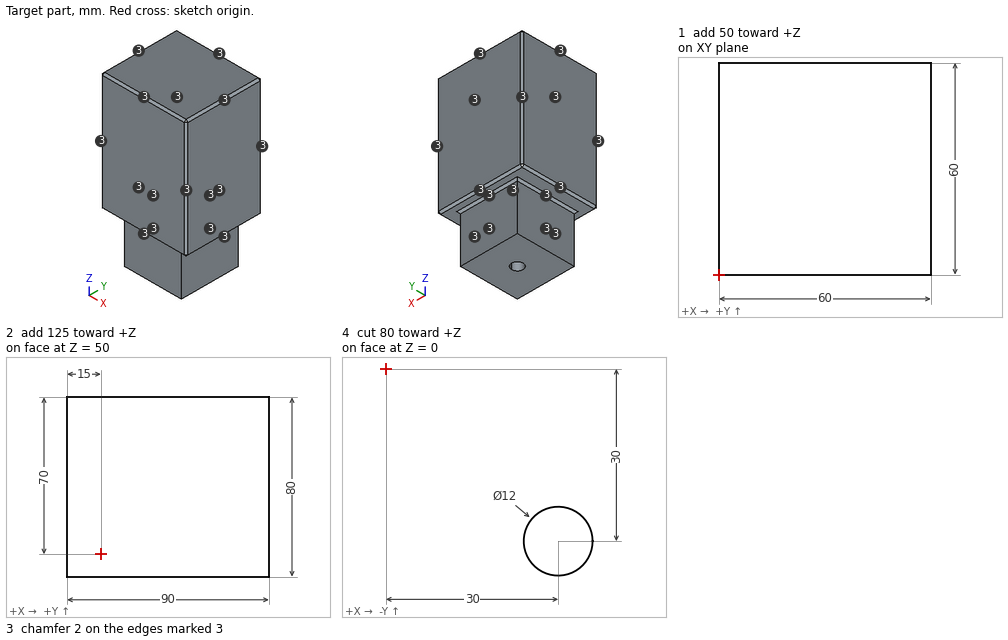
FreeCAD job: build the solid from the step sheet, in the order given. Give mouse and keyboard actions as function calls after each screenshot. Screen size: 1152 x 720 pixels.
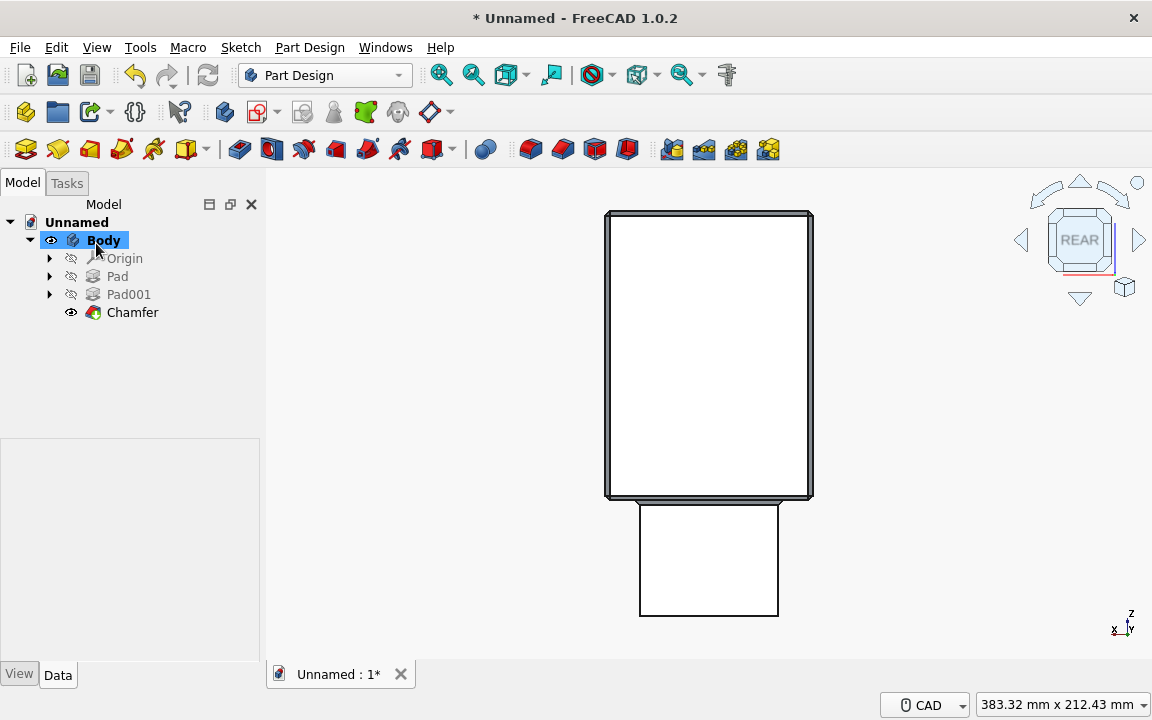
key(5)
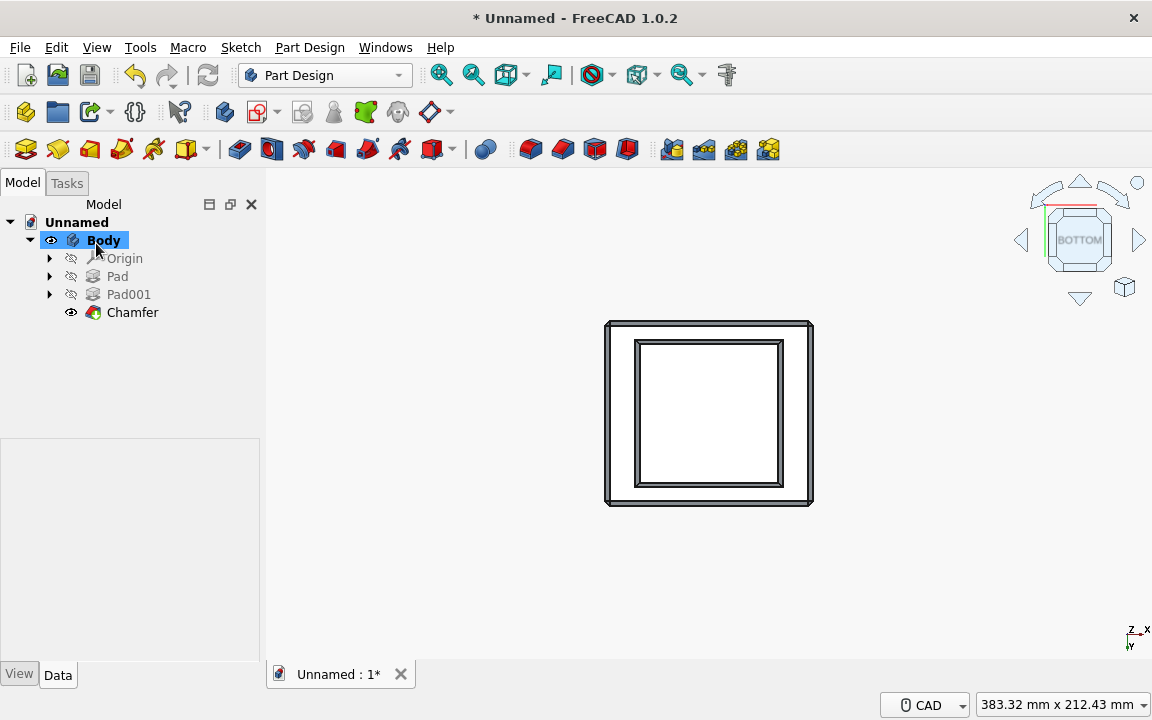
key(v)
key(f)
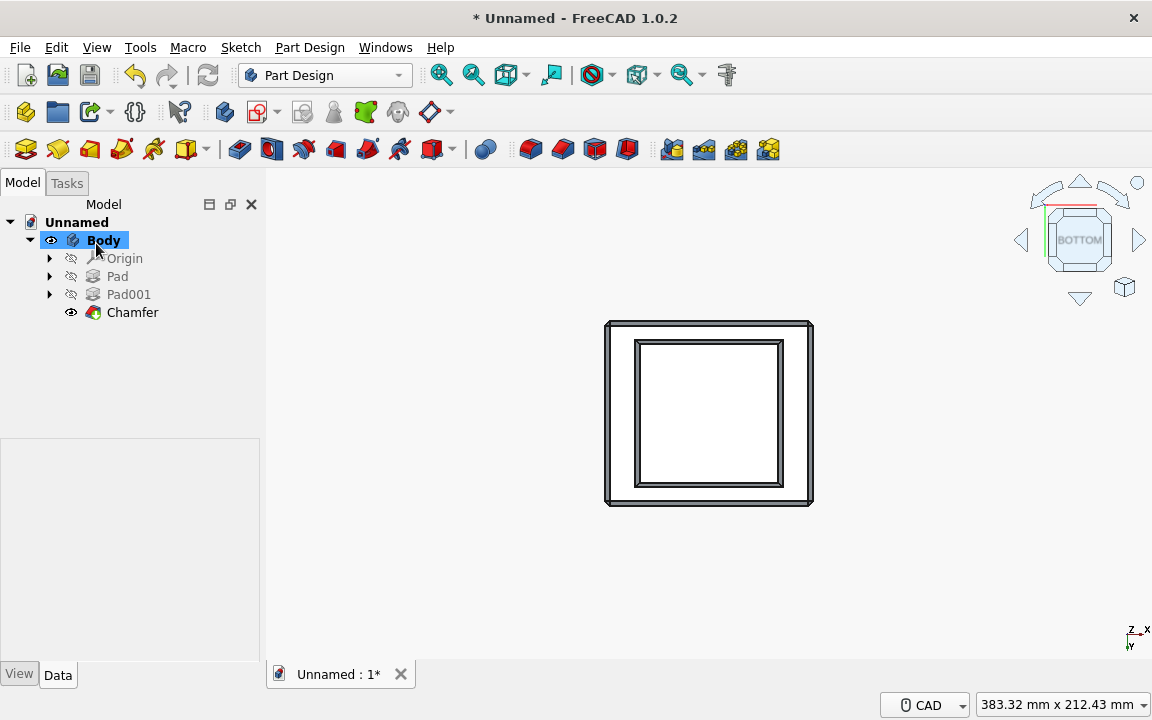
click(709, 412)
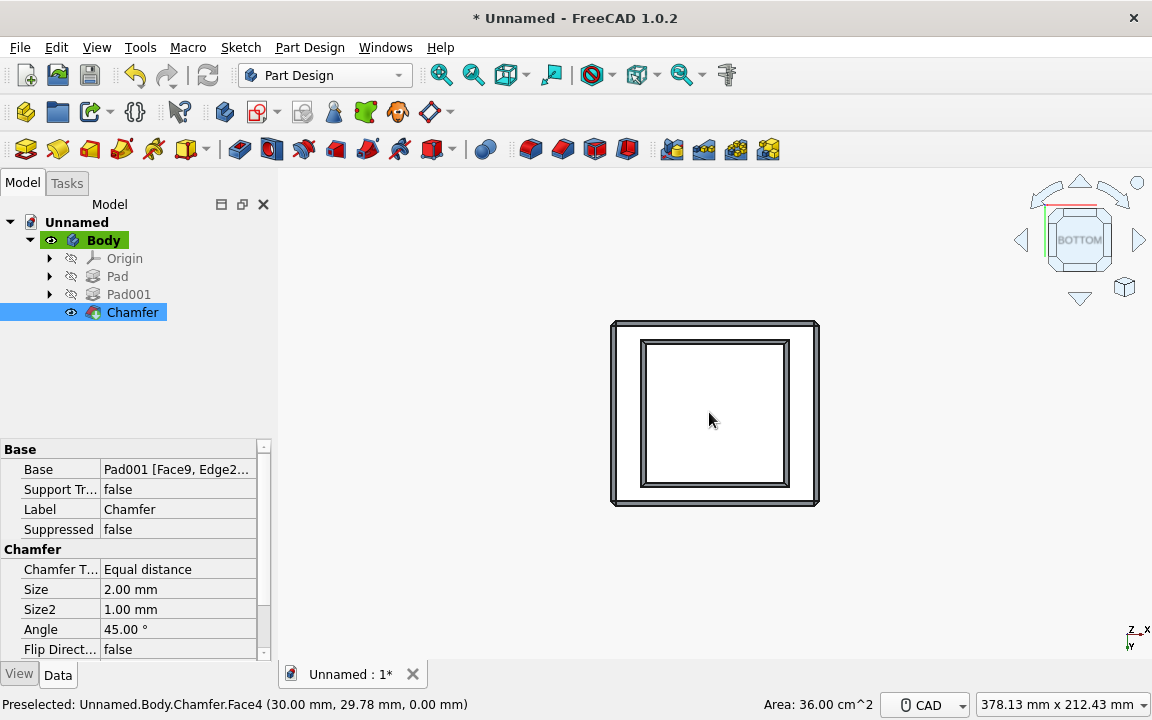
click(258, 112)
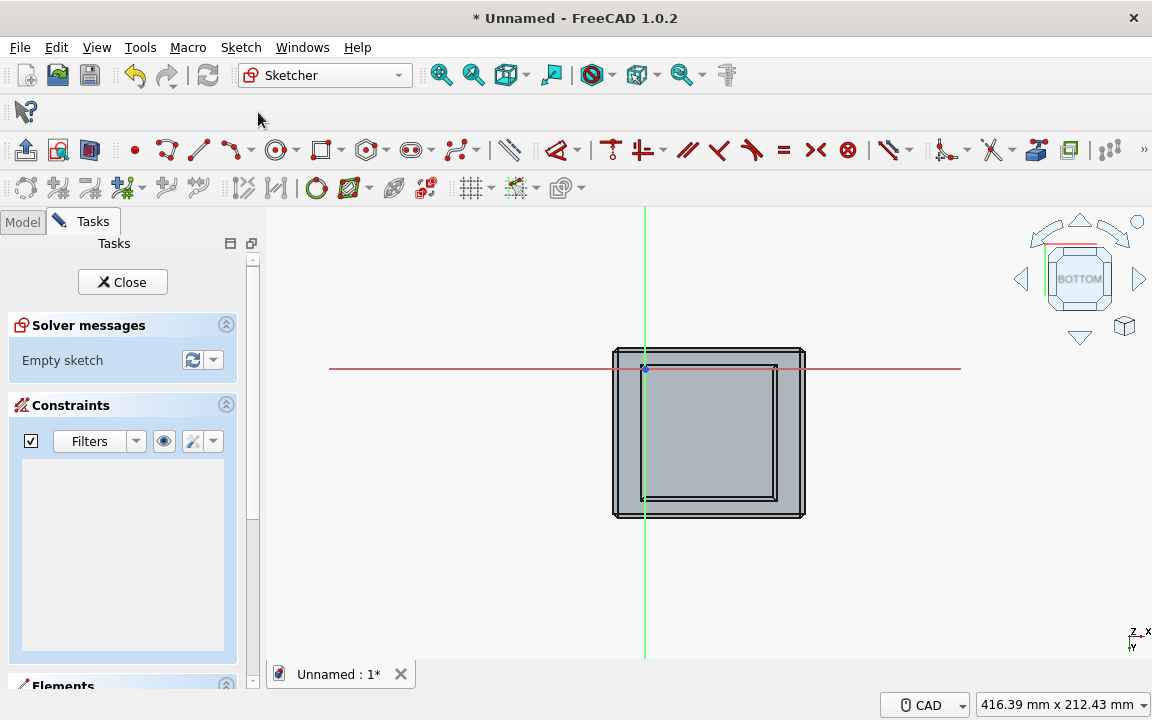
scroll(716, 433, up, 12)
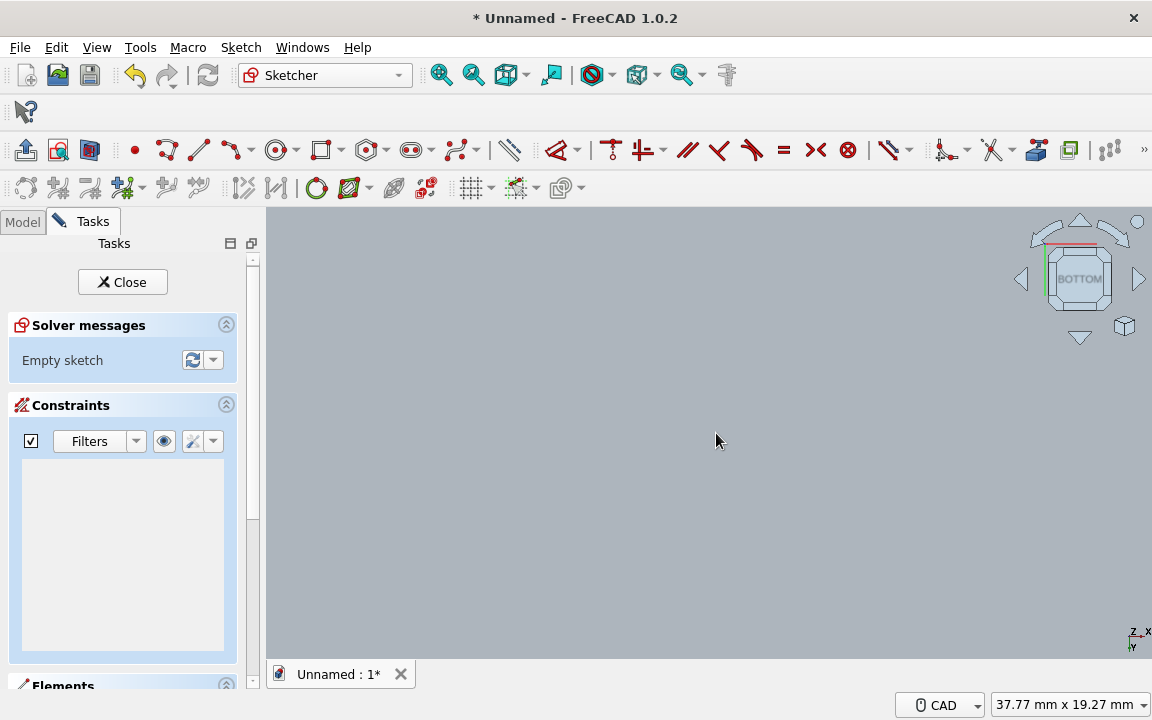
key(g)
key(c)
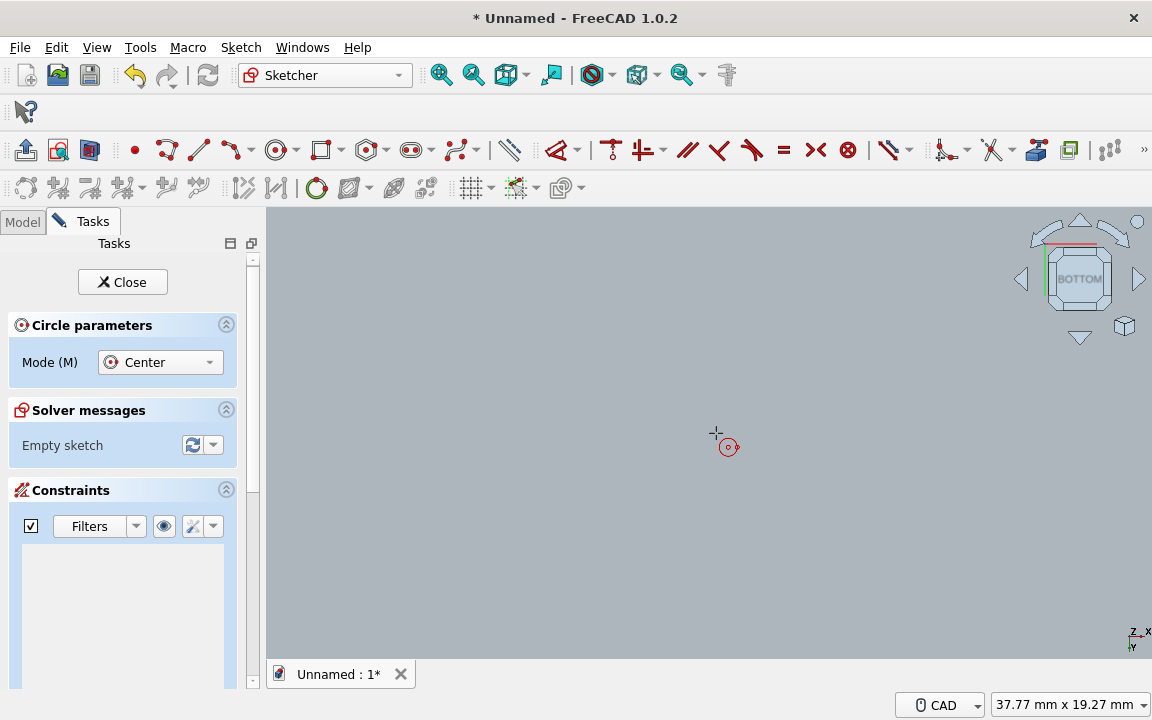
click(634, 428)
move(733, 328)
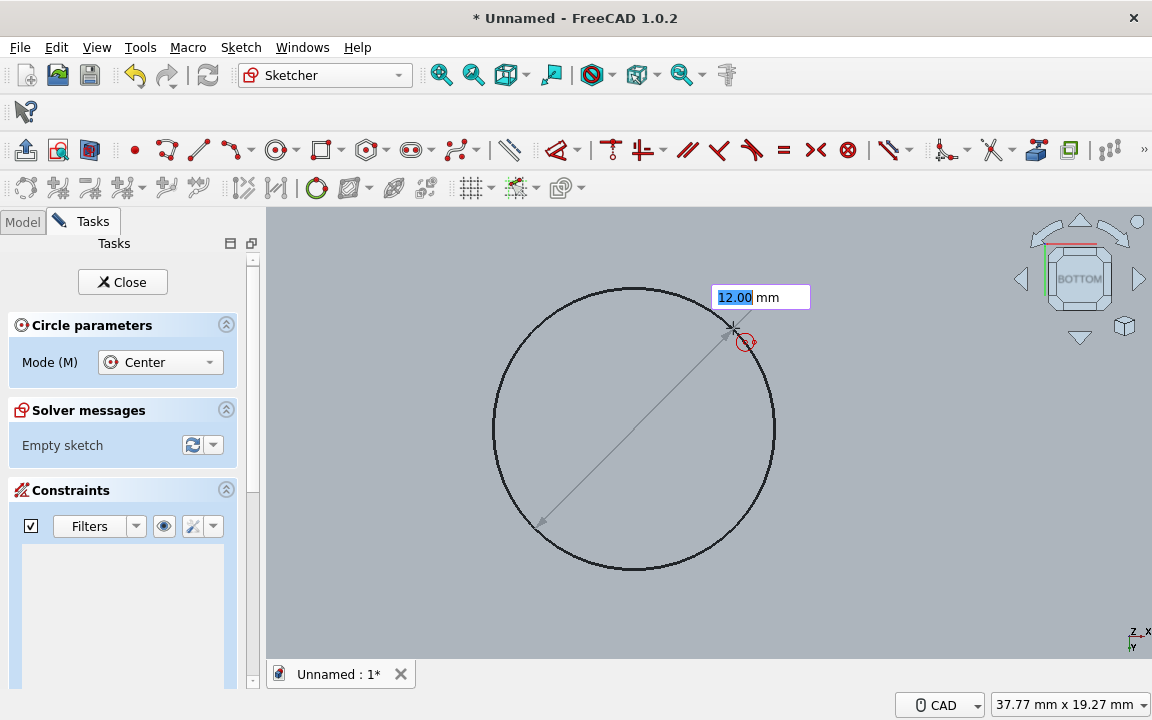
text(12)
key(Return)
key(Escape)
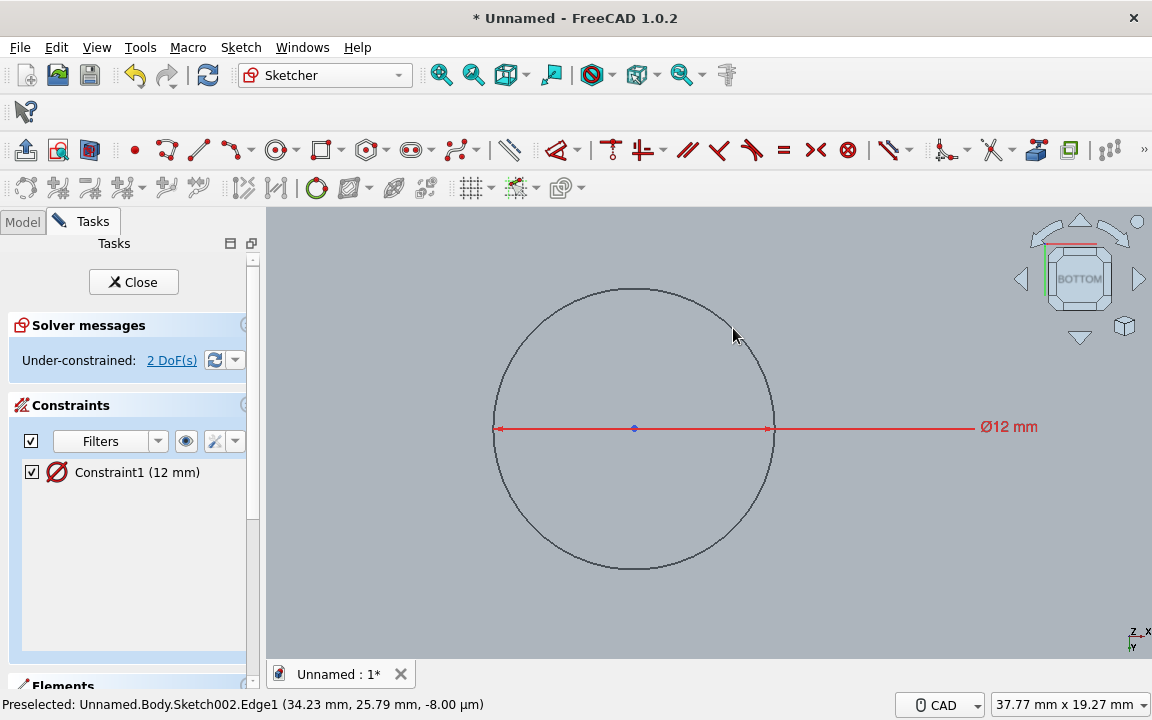
click(634, 429)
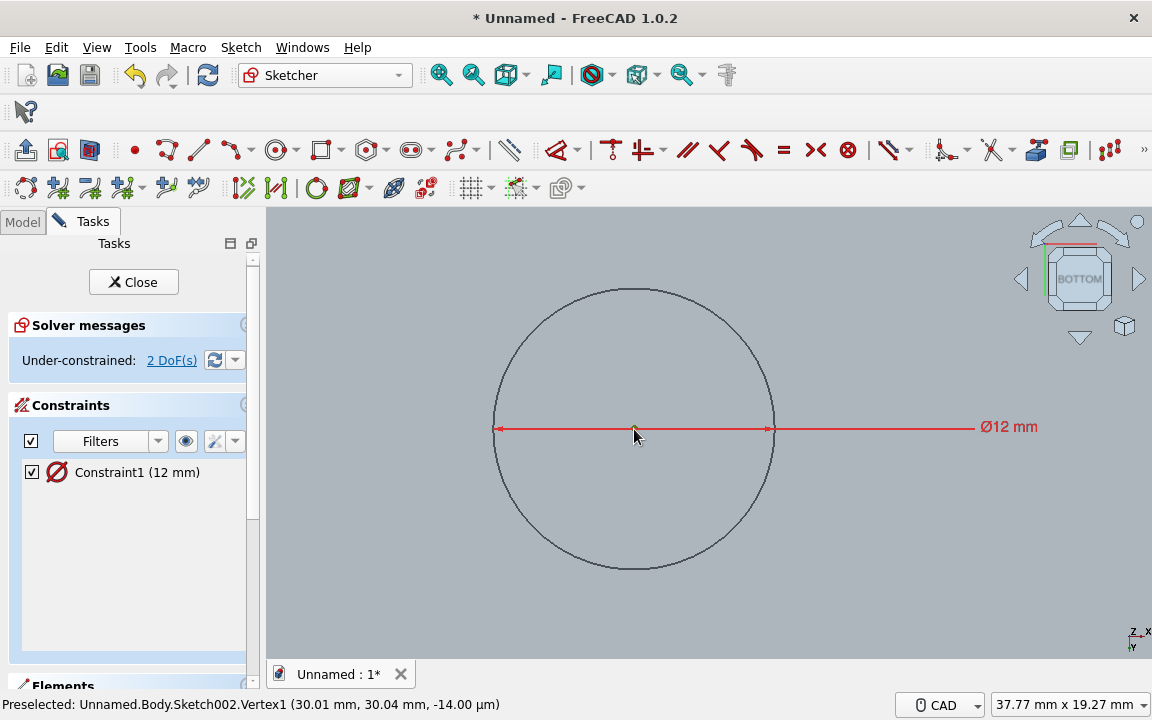
key(l)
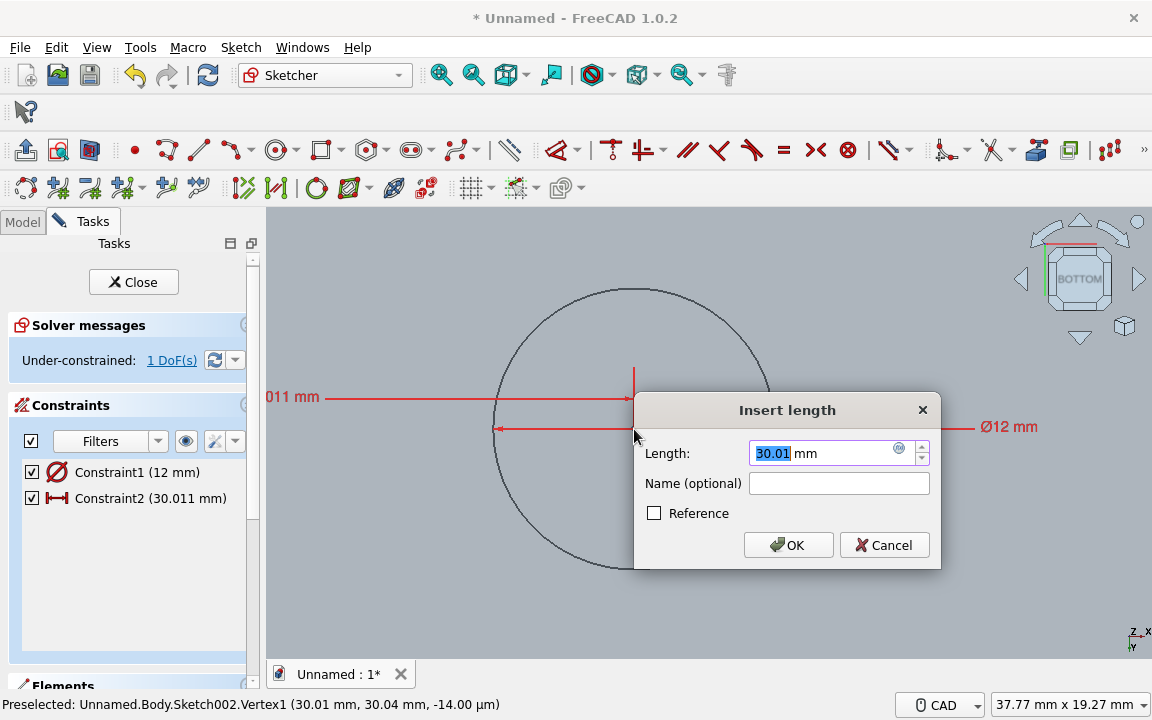
text(30)
key(Return)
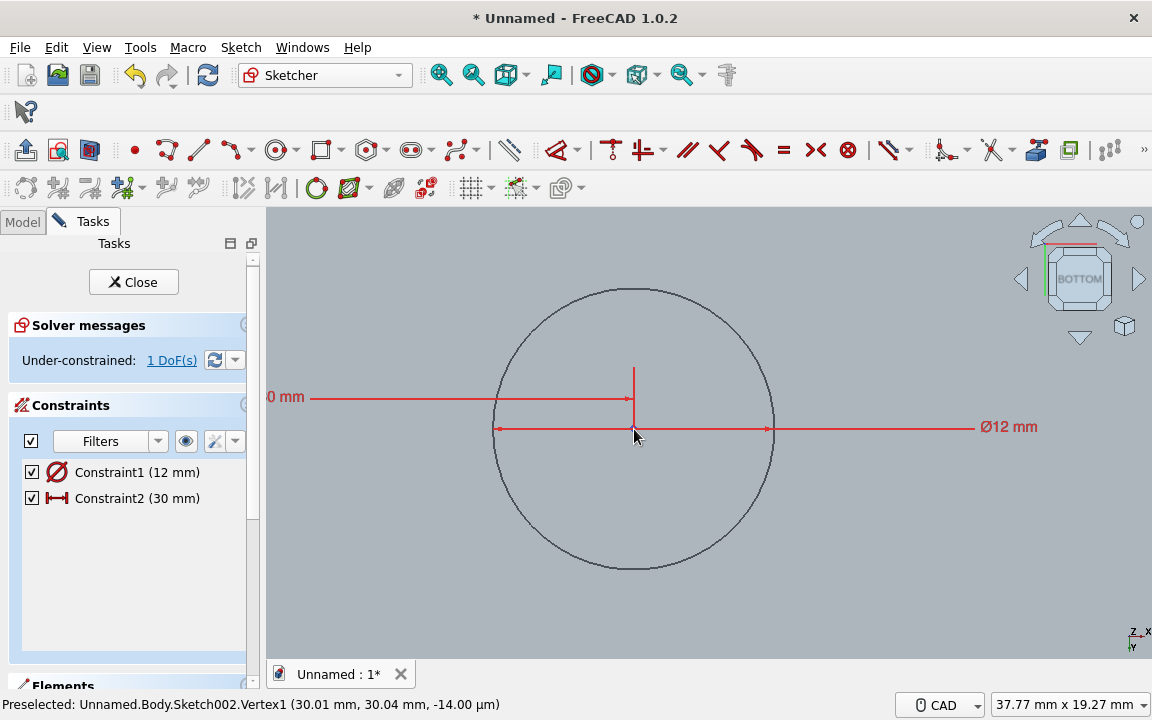
click(634, 429)